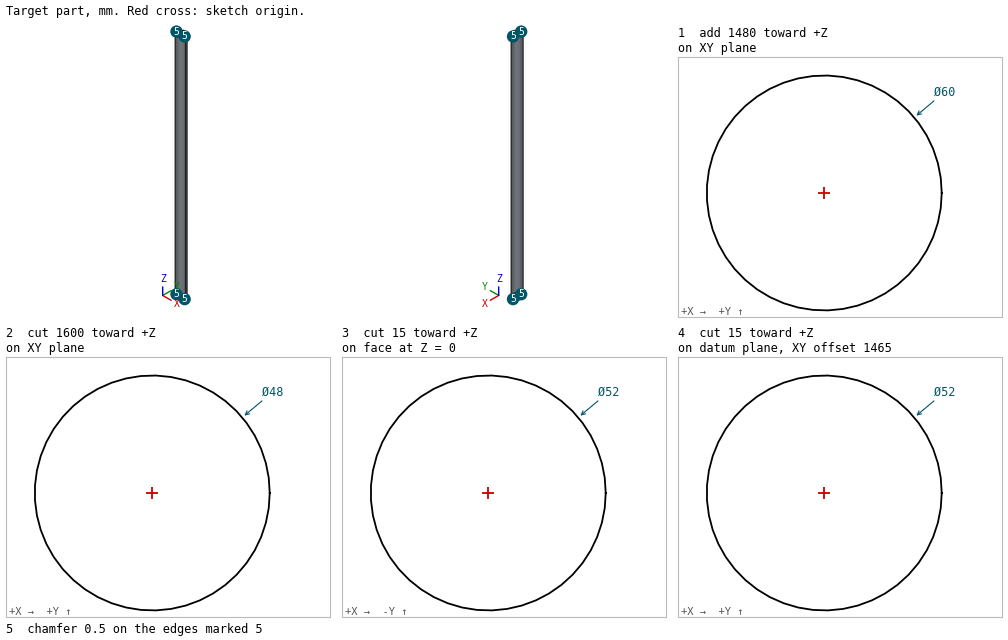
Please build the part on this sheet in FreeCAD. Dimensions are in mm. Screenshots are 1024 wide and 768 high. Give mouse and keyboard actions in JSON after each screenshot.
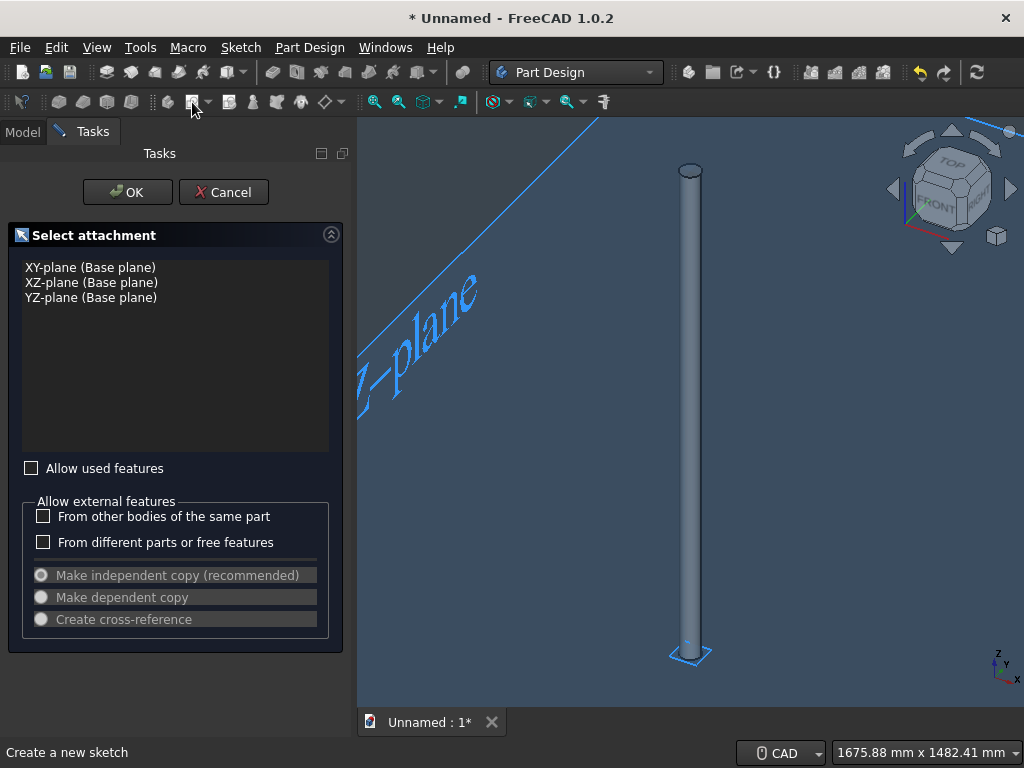
{"action": "left_click", "coordinate": [82, 268]}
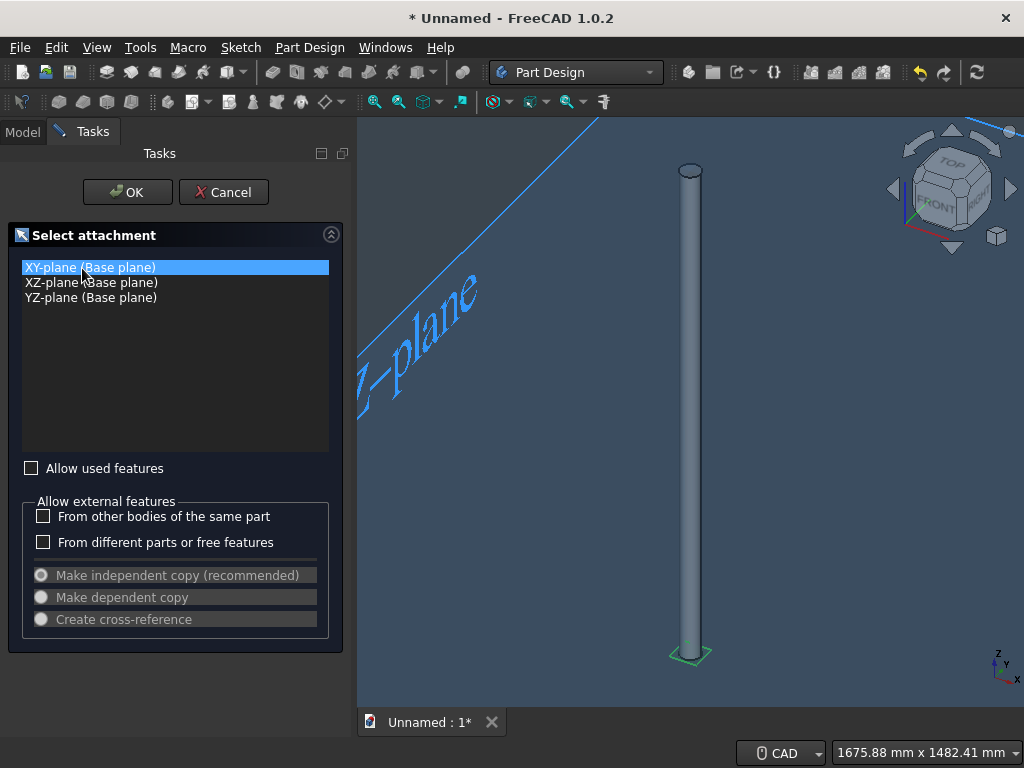
{"action": "left_click", "coordinate": [128, 192]}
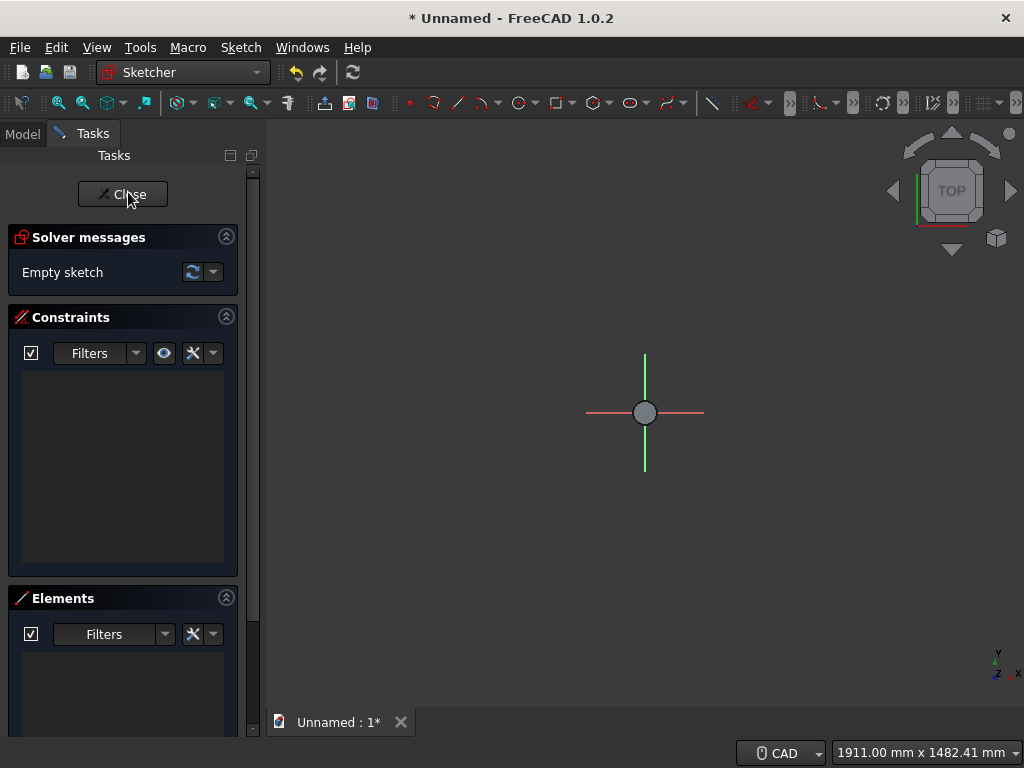
{"action": "left_click", "coordinate": [374, 104]}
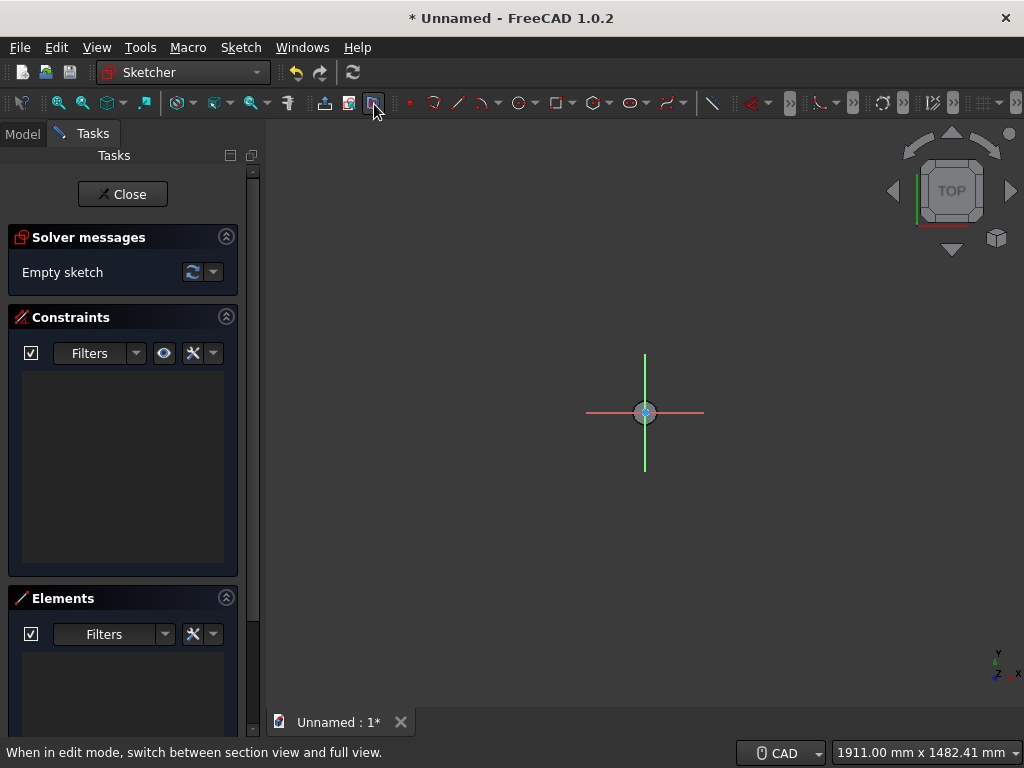
{"action": "scroll", "coordinate": [649, 413], "scroll_direction": "up", "scroll_amount": 15}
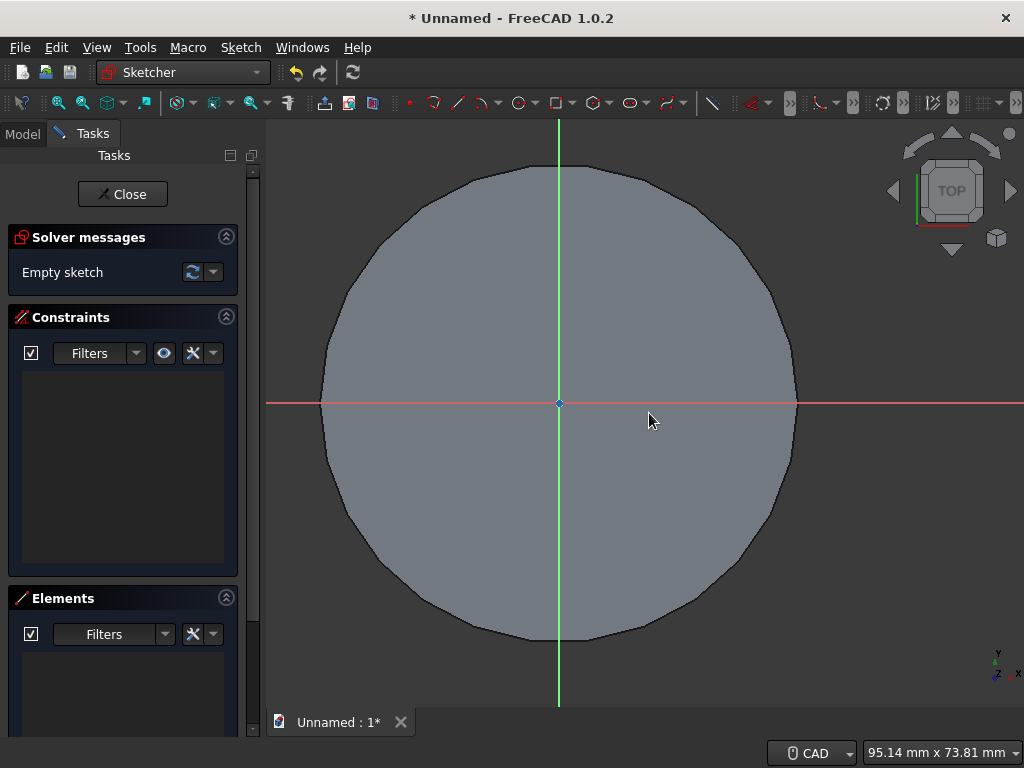
{"action": "left_click", "coordinate": [520, 104]}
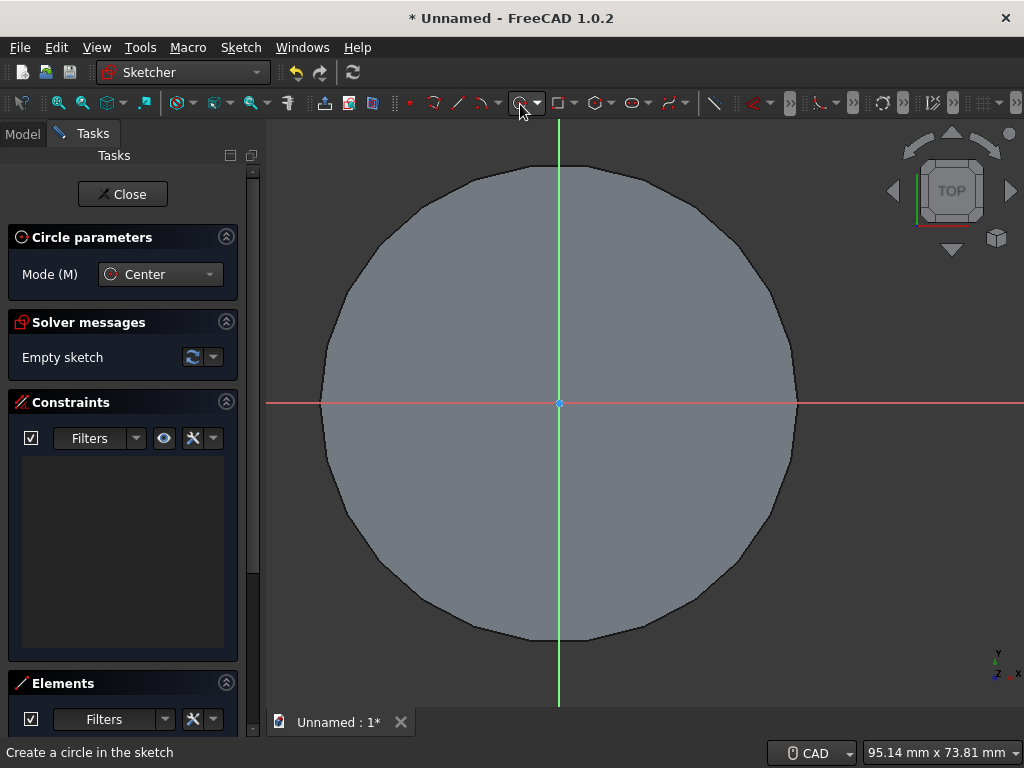
{"action": "left_click", "coordinate": [559, 403]}
{"action": "mouse_move", "coordinate": [694, 268]}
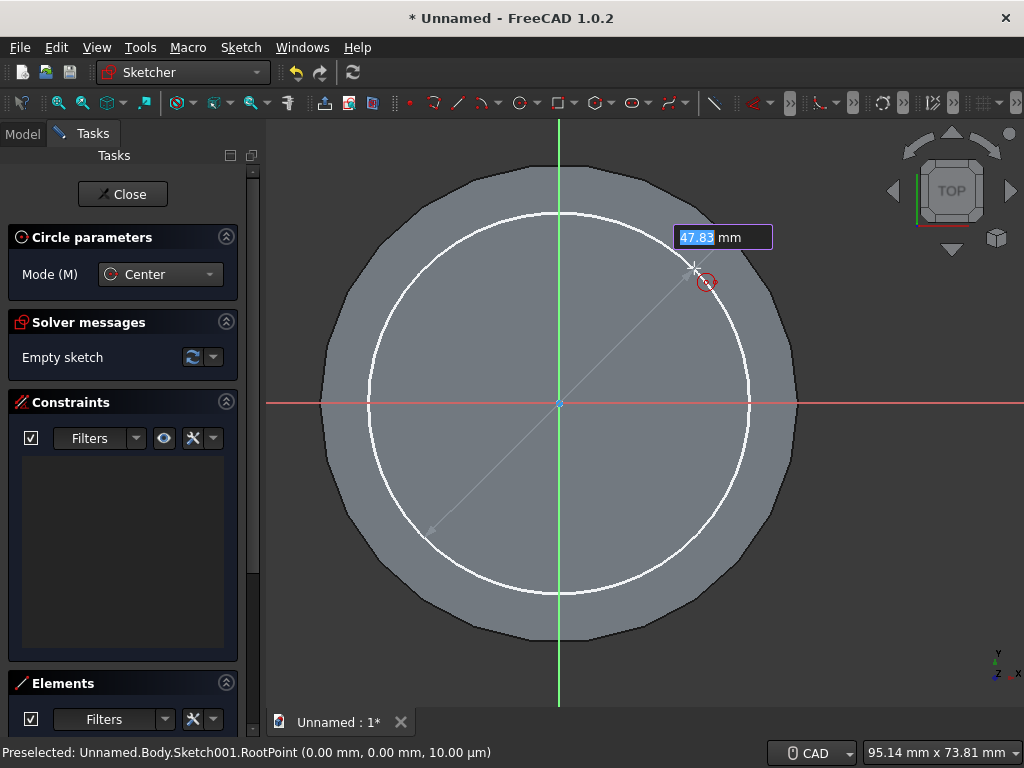
{"action": "type", "text": "48"}
{"action": "key", "text": "Return"}
{"action": "key", "text": "Escape"}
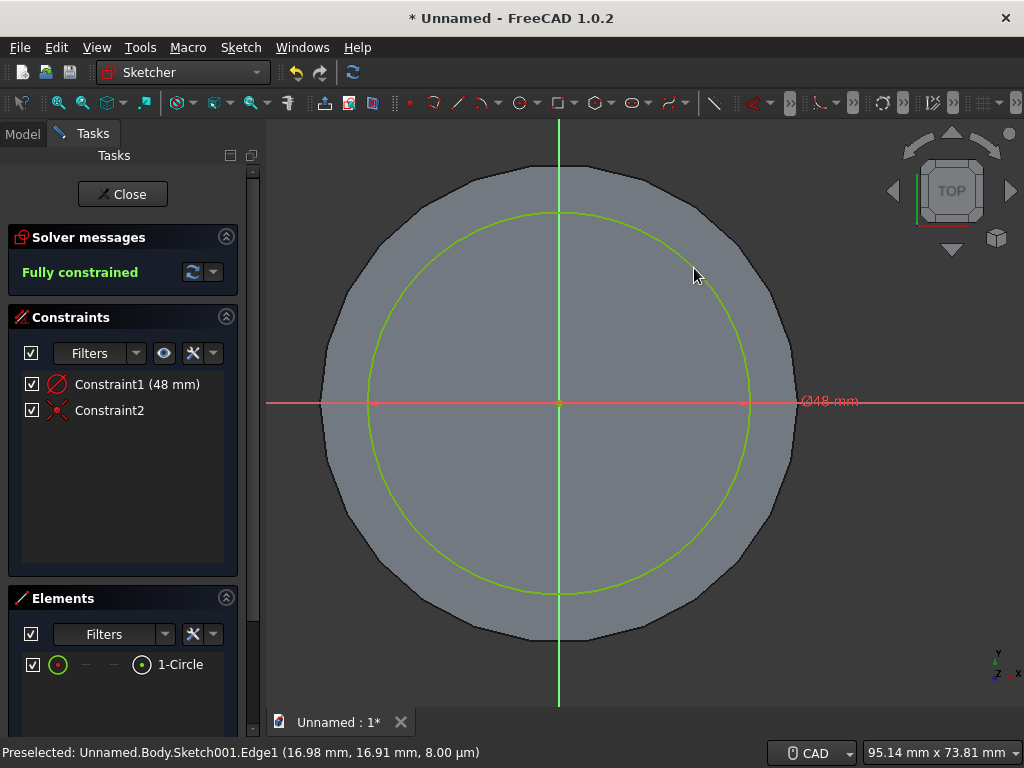
{"action": "left_click", "coordinate": [123, 194]}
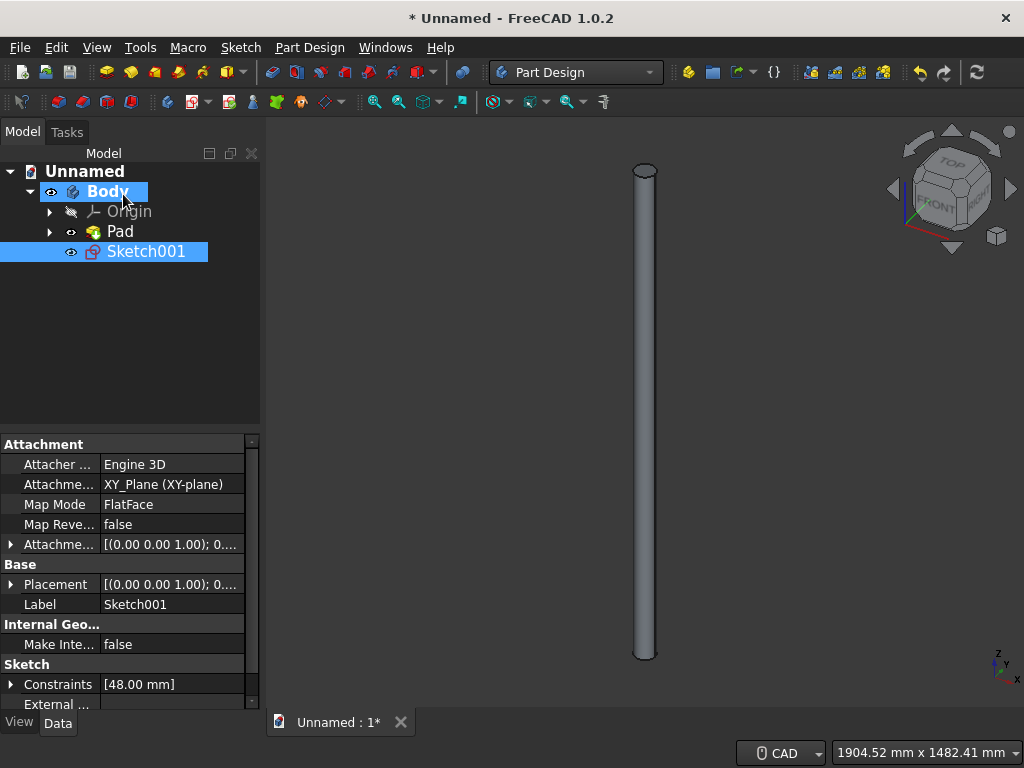
{"action": "left_click", "coordinate": [274, 72]}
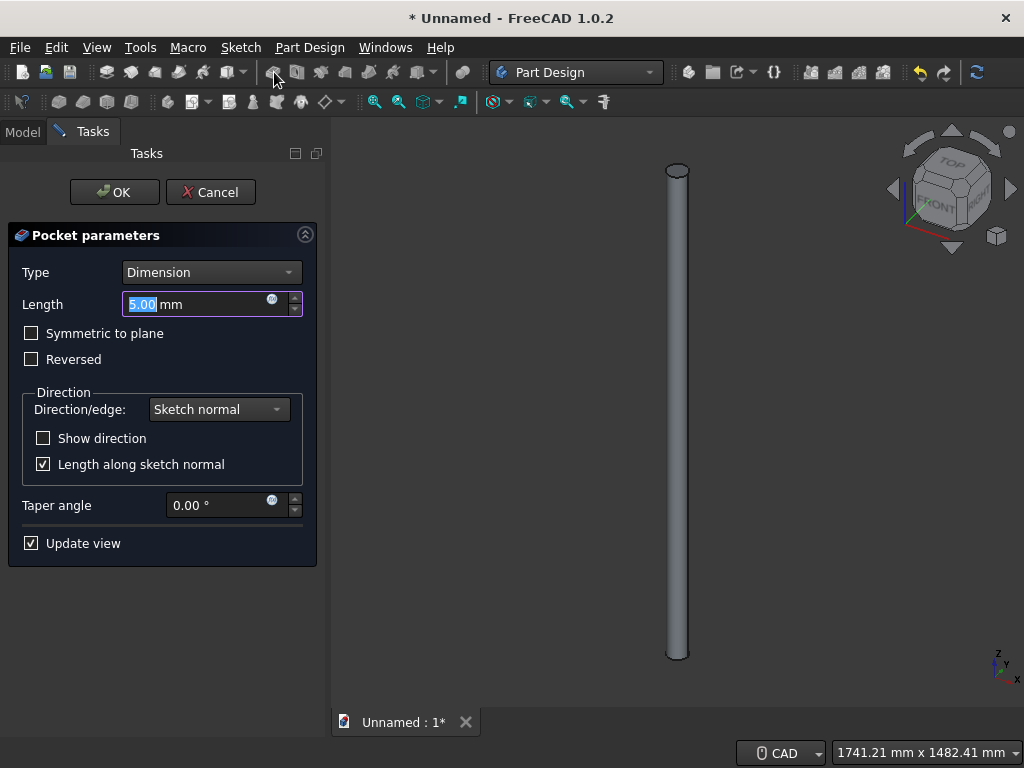
{"action": "type", "text": "1600"}
{"action": "key", "text": "Tab"}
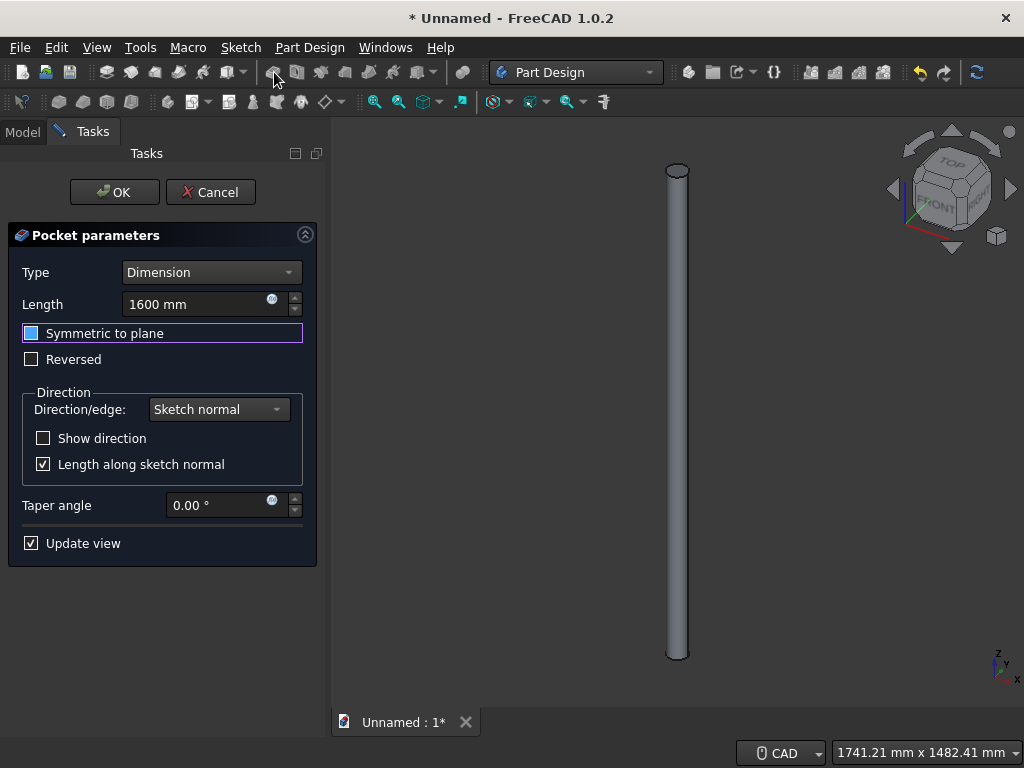
{"action": "left_click", "coordinate": [30, 359]}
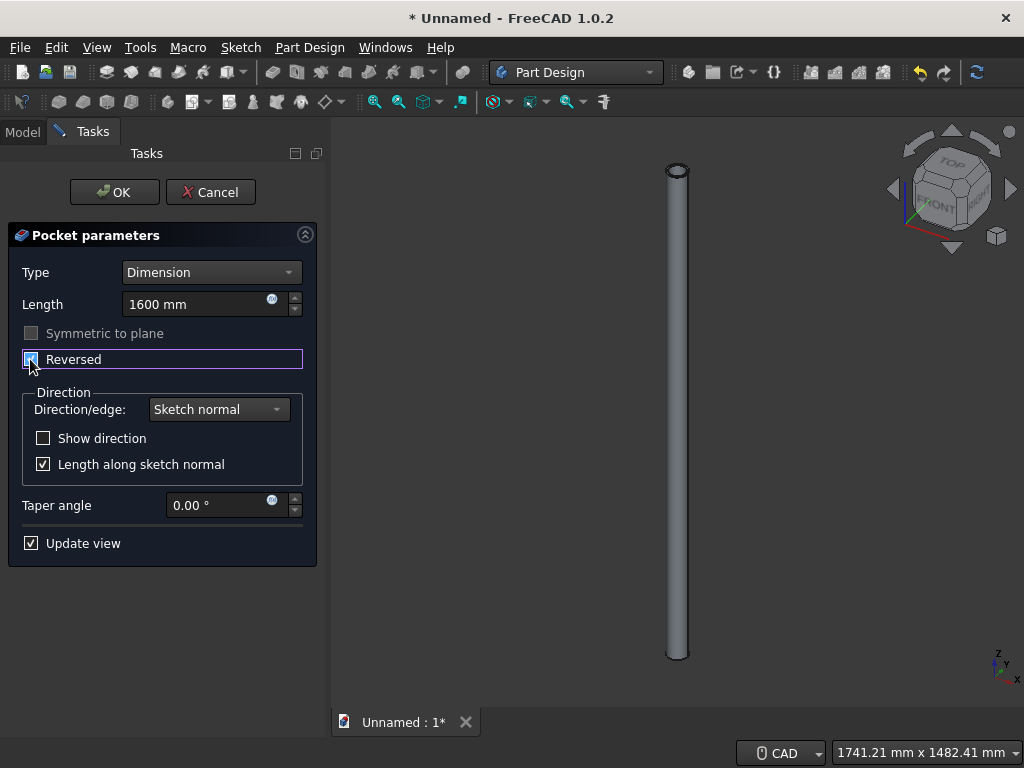
{"action": "left_click", "coordinate": [115, 192]}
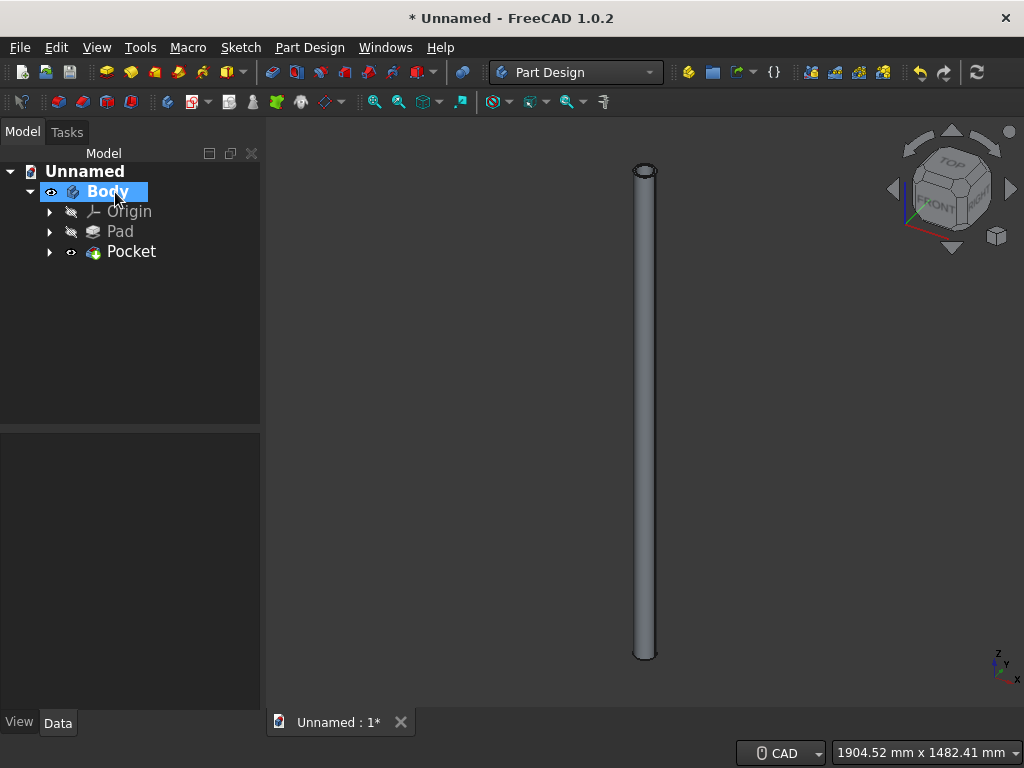
{"action": "key", "text": "5"}